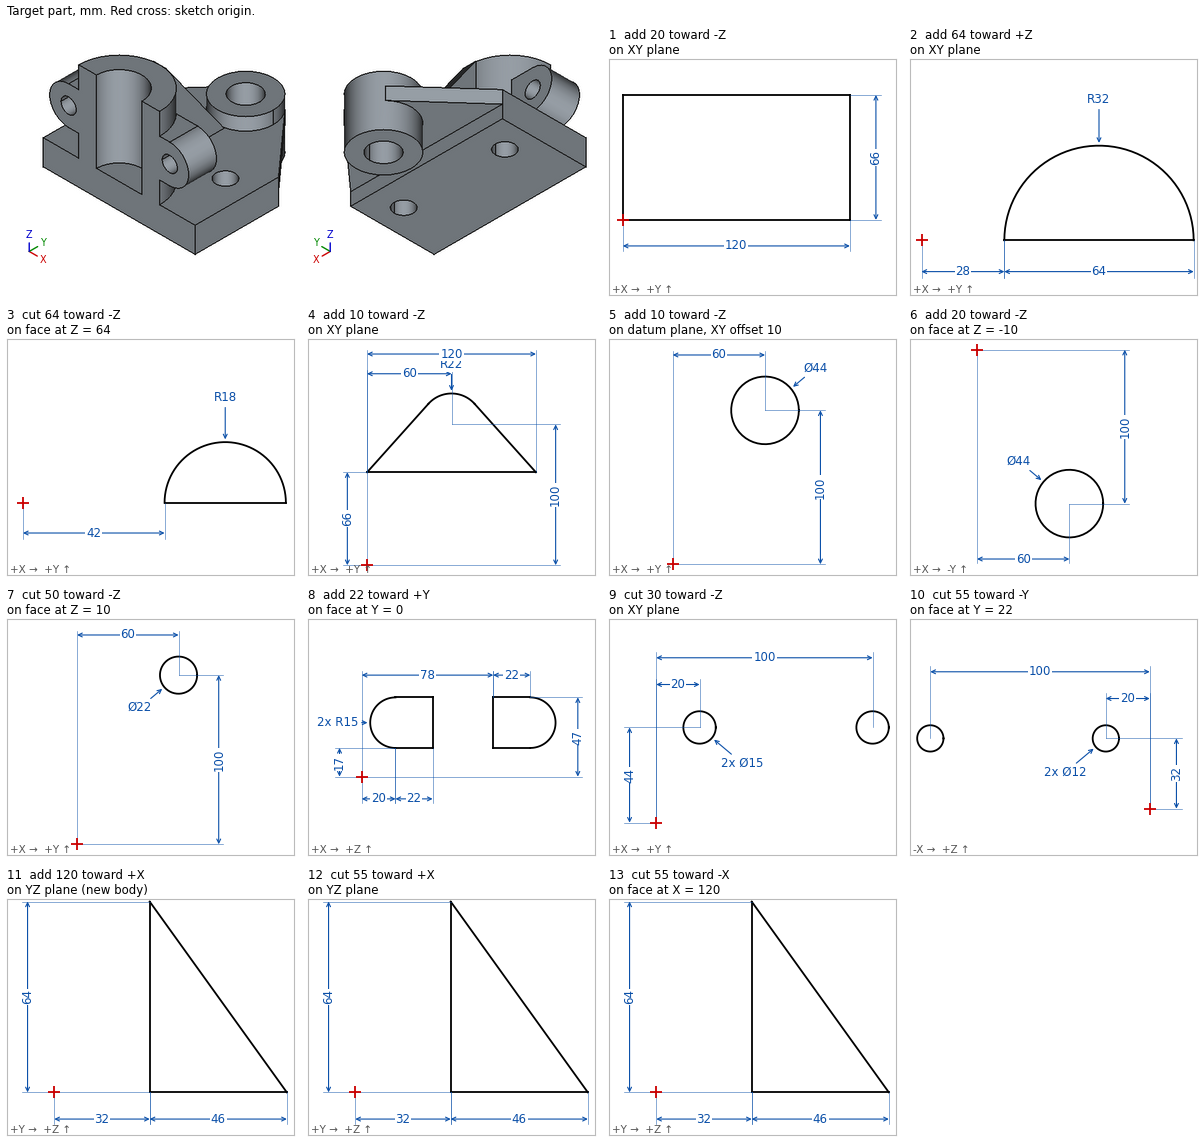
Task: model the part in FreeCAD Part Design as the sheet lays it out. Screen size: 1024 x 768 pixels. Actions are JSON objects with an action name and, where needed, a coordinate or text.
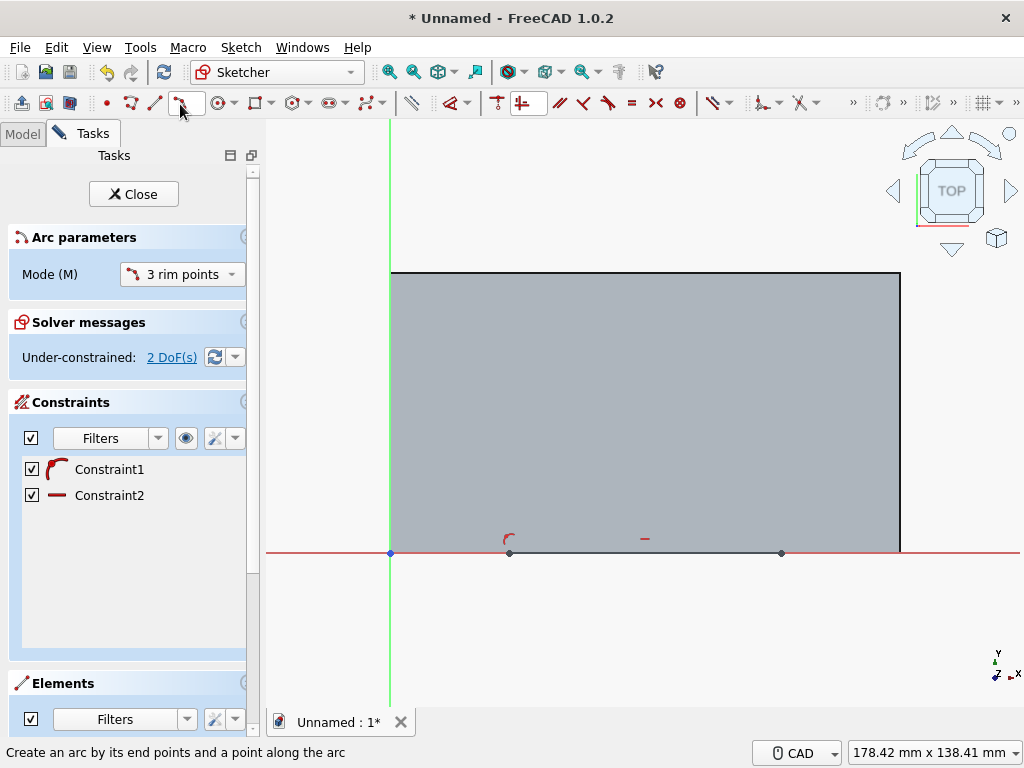
{"action": "left_click", "coordinate": [781, 544]}
{"action": "left_click", "coordinate": [509, 553]}
{"action": "left_click", "coordinate": [645, 417]}
{"action": "key", "text": "Escape"}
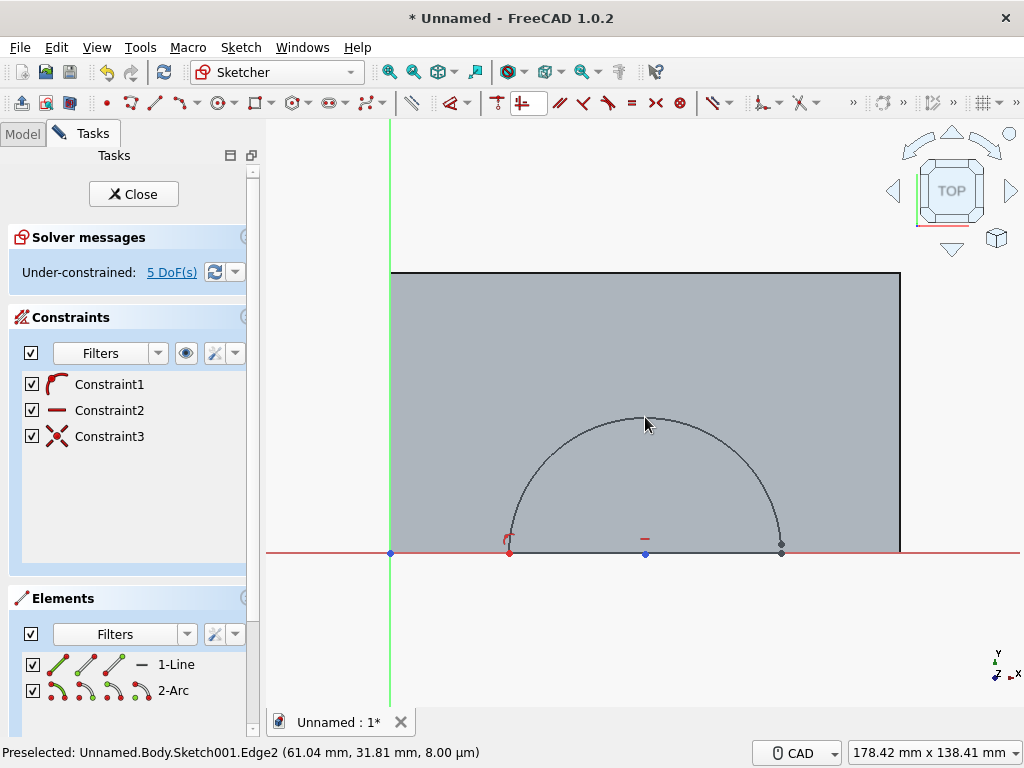
{"action": "left_click", "coordinate": [645, 554]}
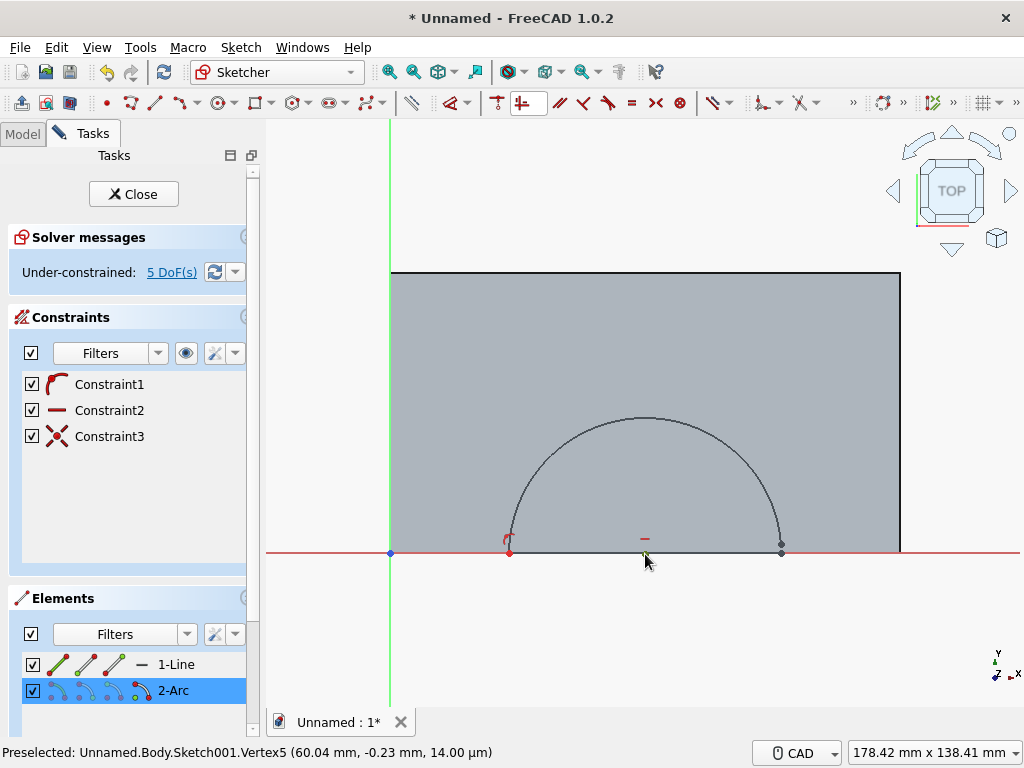
{"action": "left_click", "coordinate": [334, 553]}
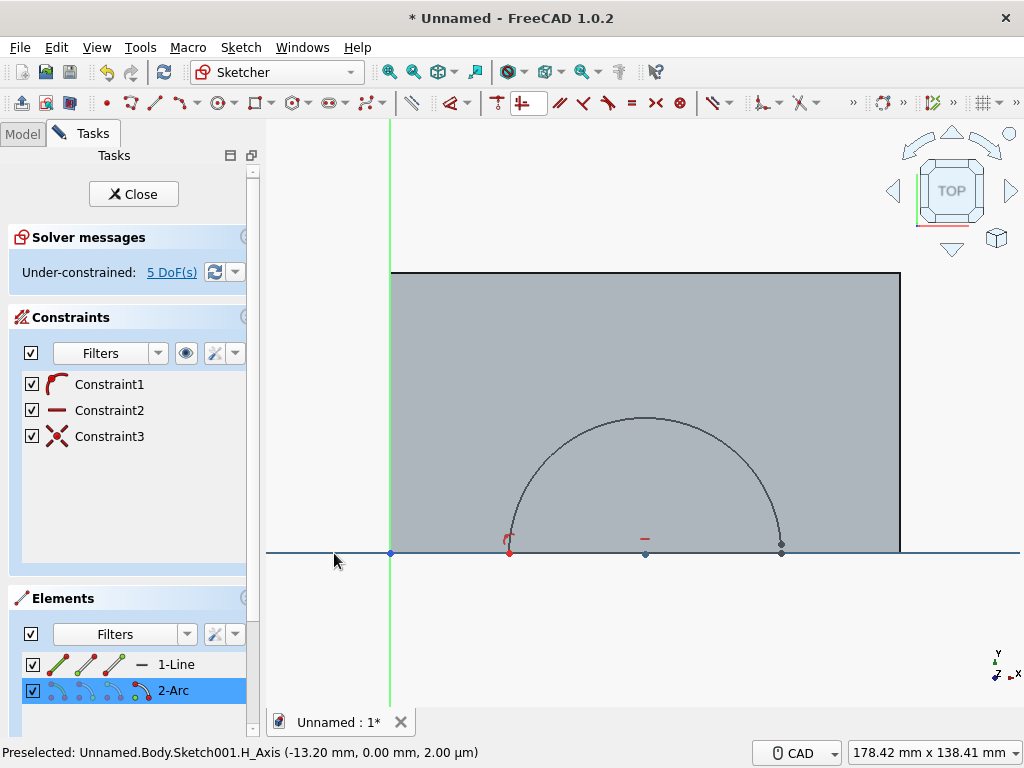
{"action": "left_click", "coordinate": [498, 104]}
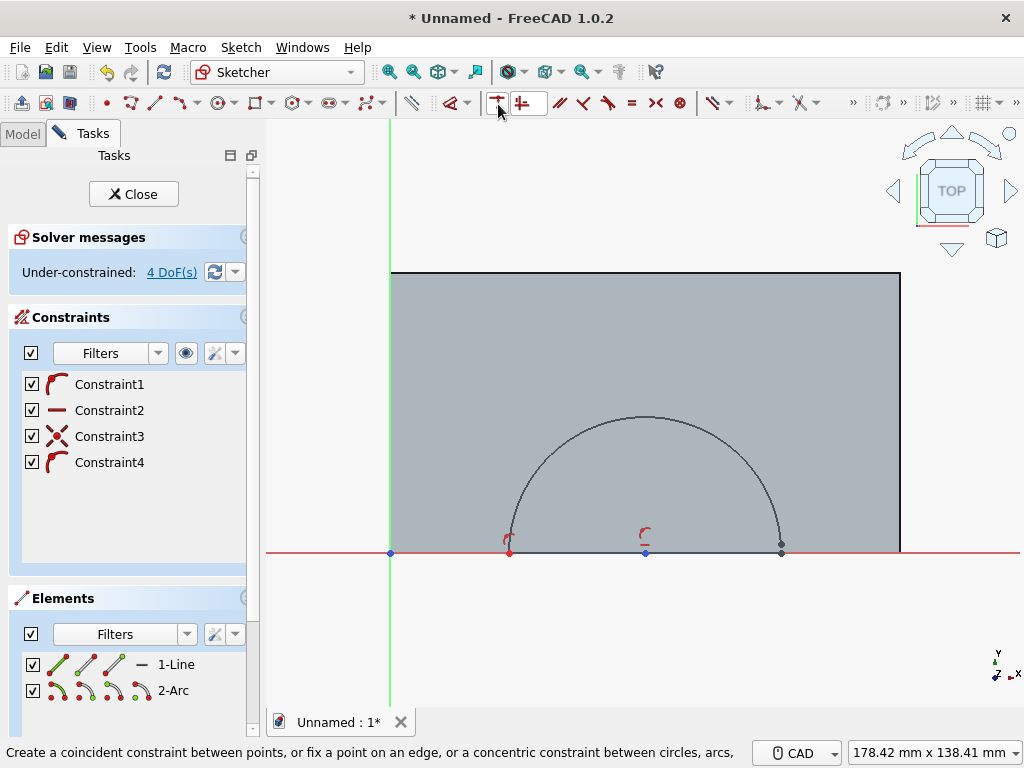
{"action": "left_click", "coordinate": [450, 104]}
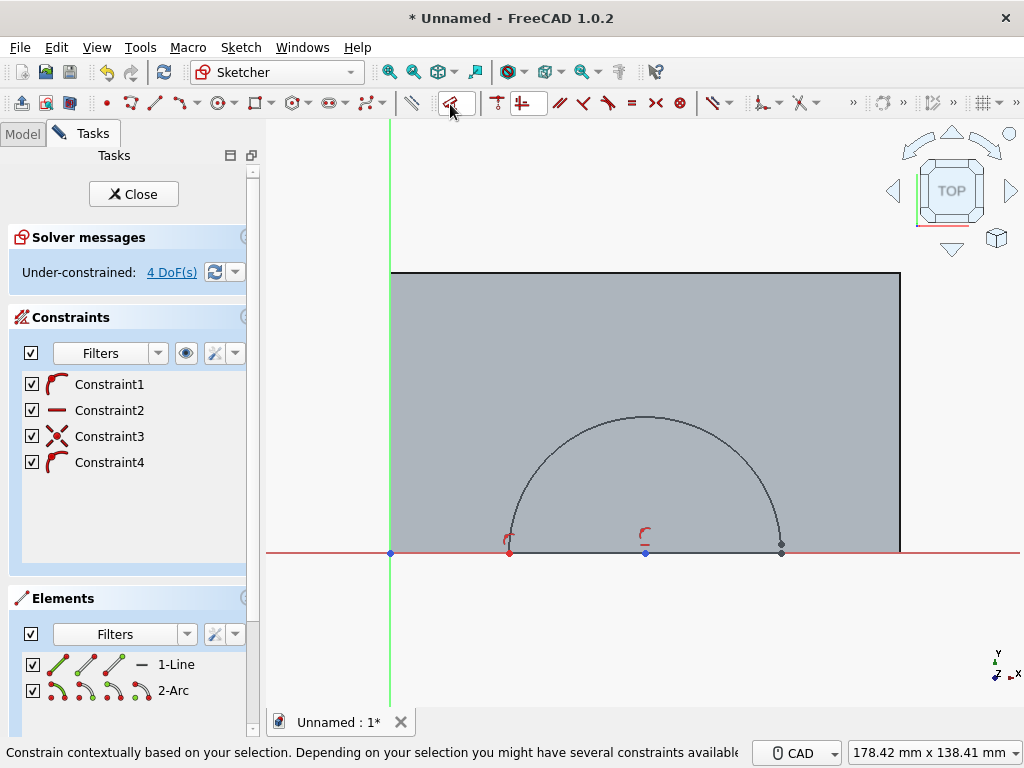
{"action": "left_click", "coordinate": [720, 440]}
{"action": "left_click", "coordinate": [738, 413]}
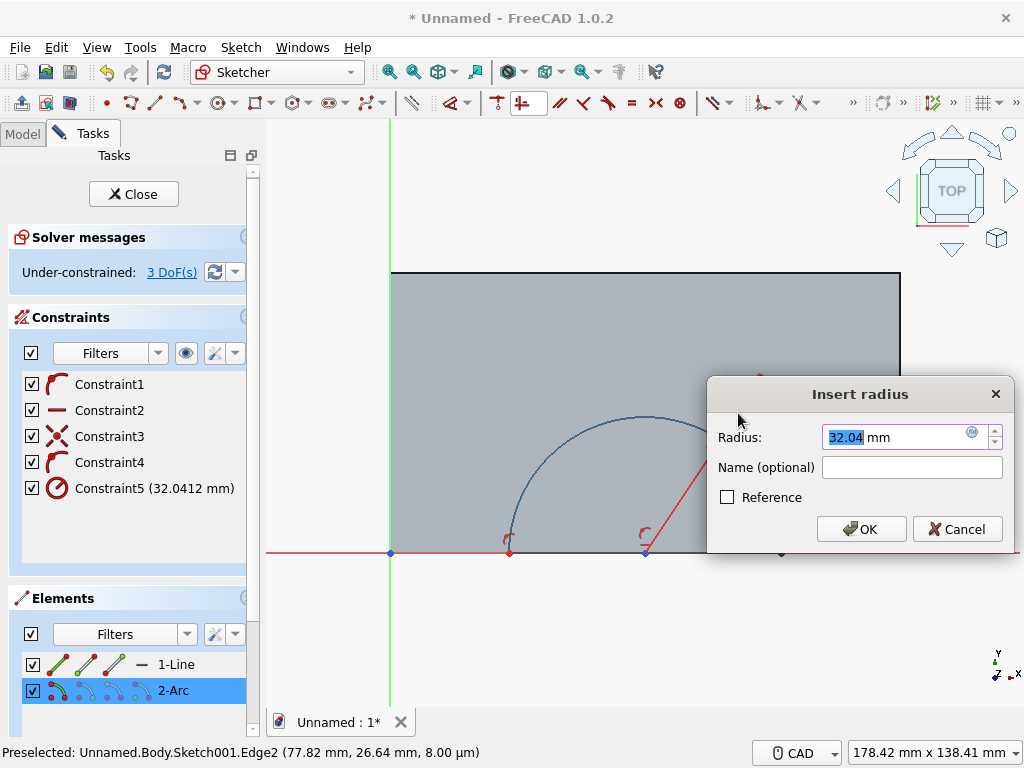
{"action": "type", "text": "32"}
{"action": "key", "text": "Return"}
{"action": "key", "text": "Escape"}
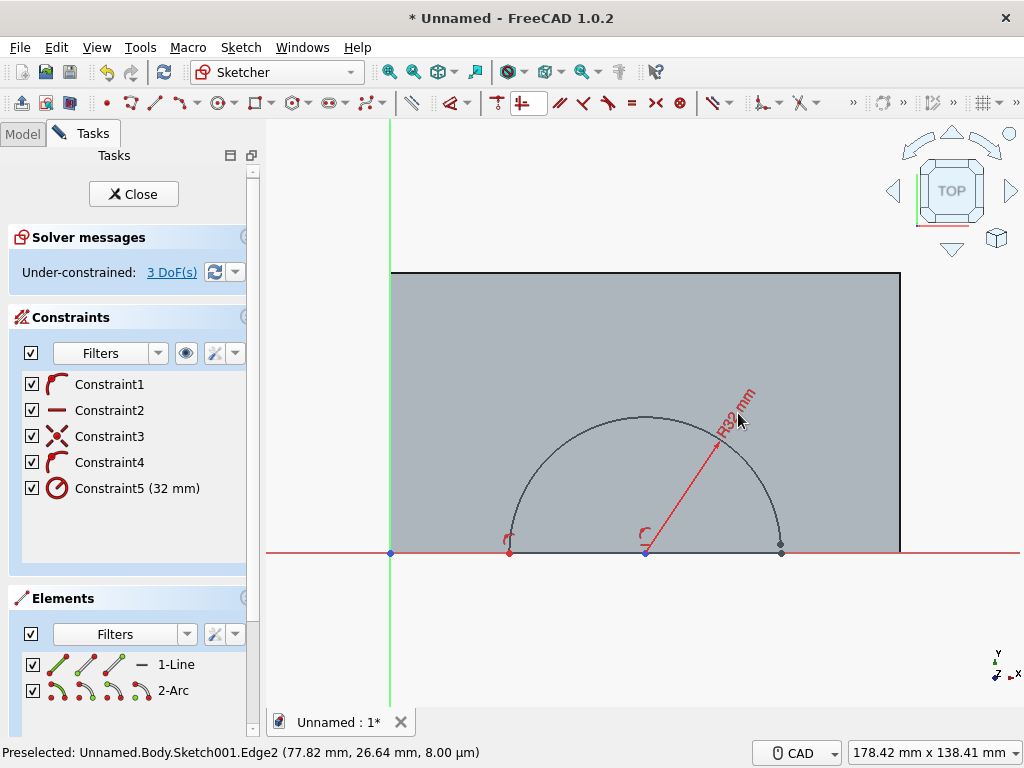
{"action": "left_click", "coordinate": [781, 545]}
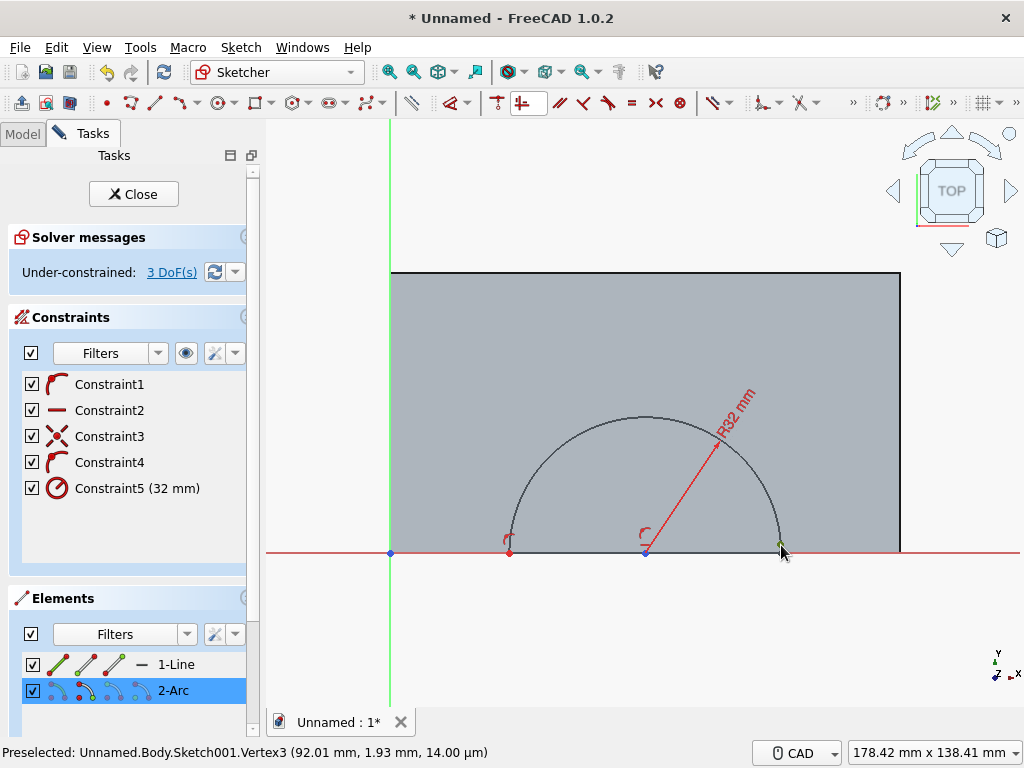
{"action": "left_click", "coordinate": [334, 553]}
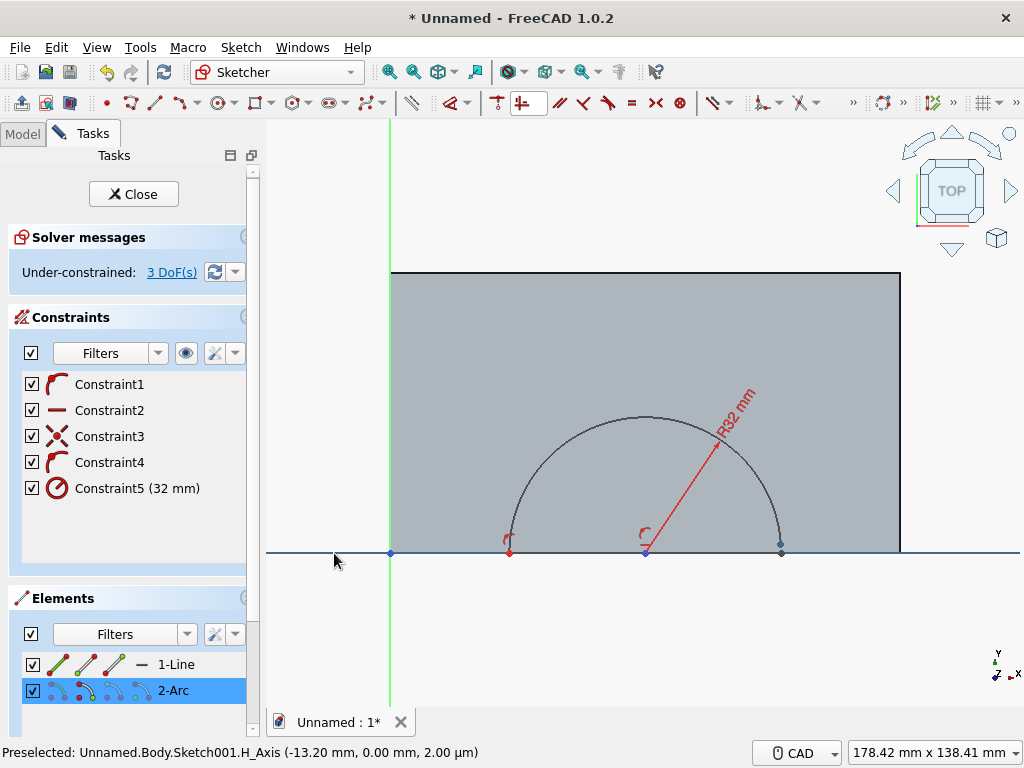
{"action": "left_click", "coordinate": [498, 104]}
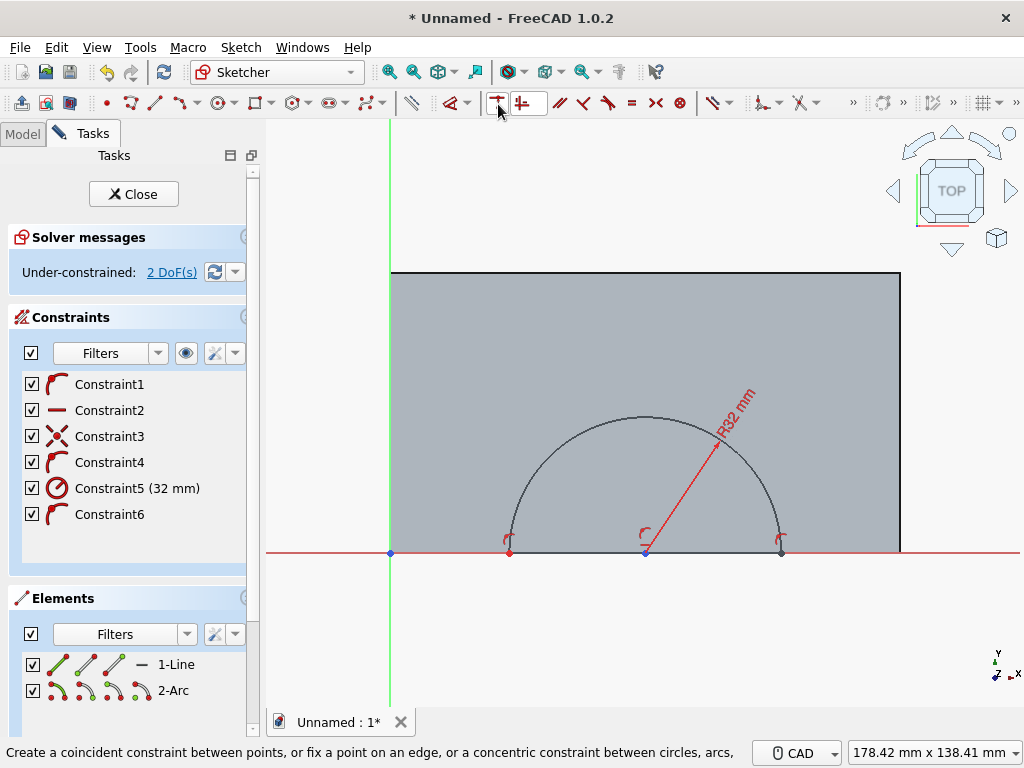
{"action": "left_click", "coordinate": [450, 104]}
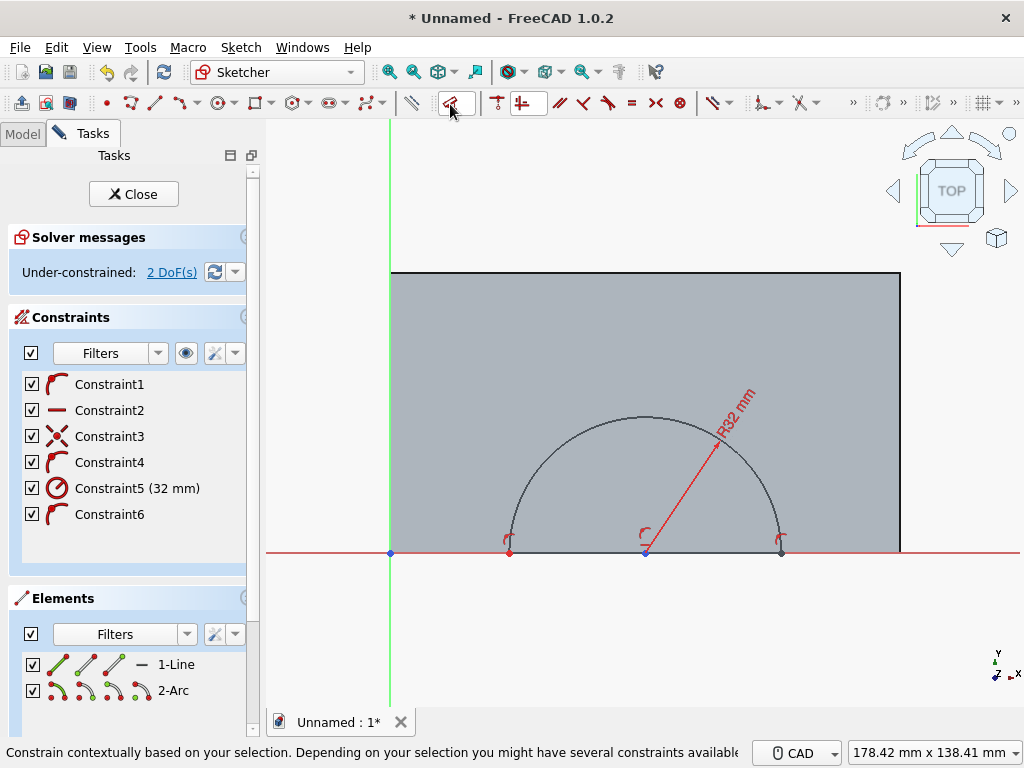
{"action": "left_click", "coordinate": [591, 553]}
{"action": "left_click", "coordinate": [645, 587]}